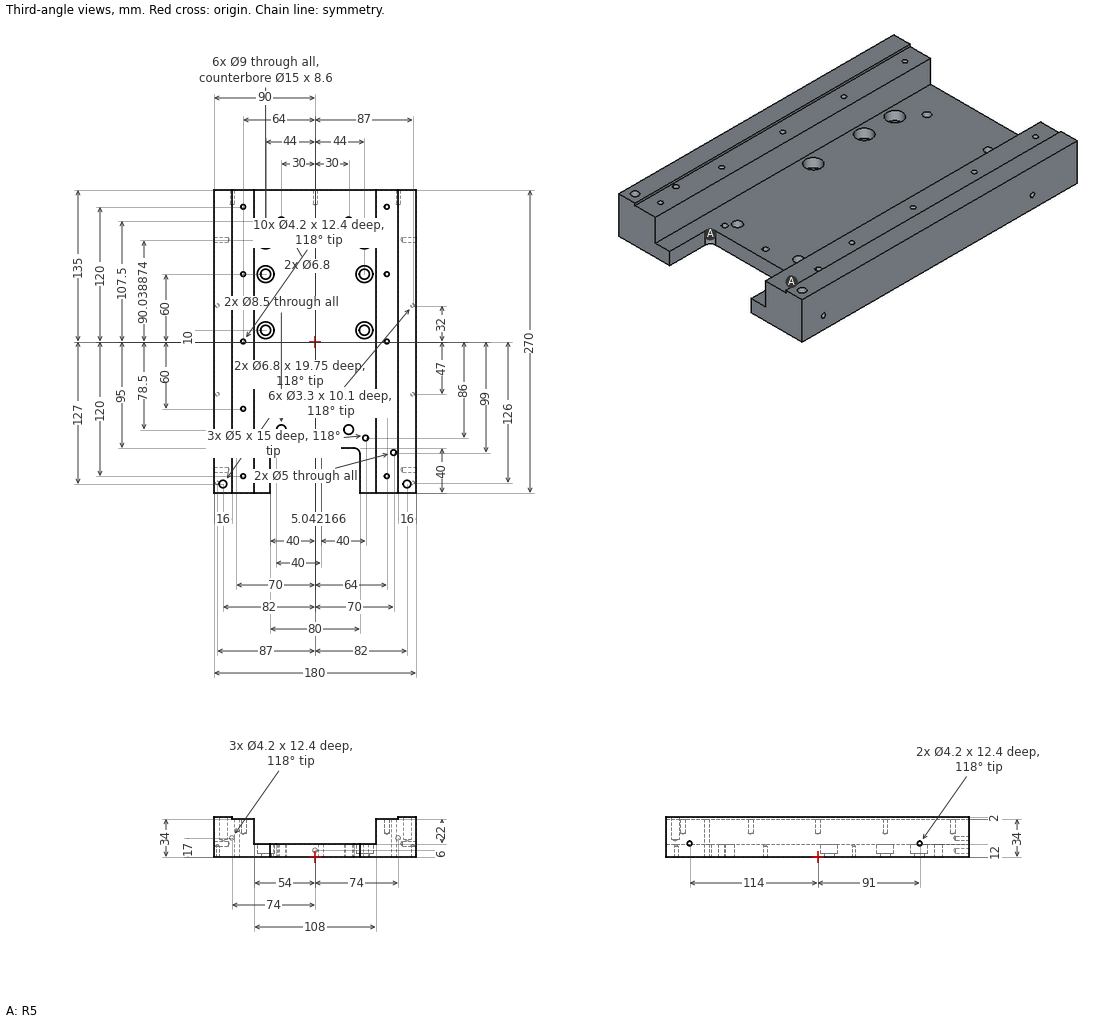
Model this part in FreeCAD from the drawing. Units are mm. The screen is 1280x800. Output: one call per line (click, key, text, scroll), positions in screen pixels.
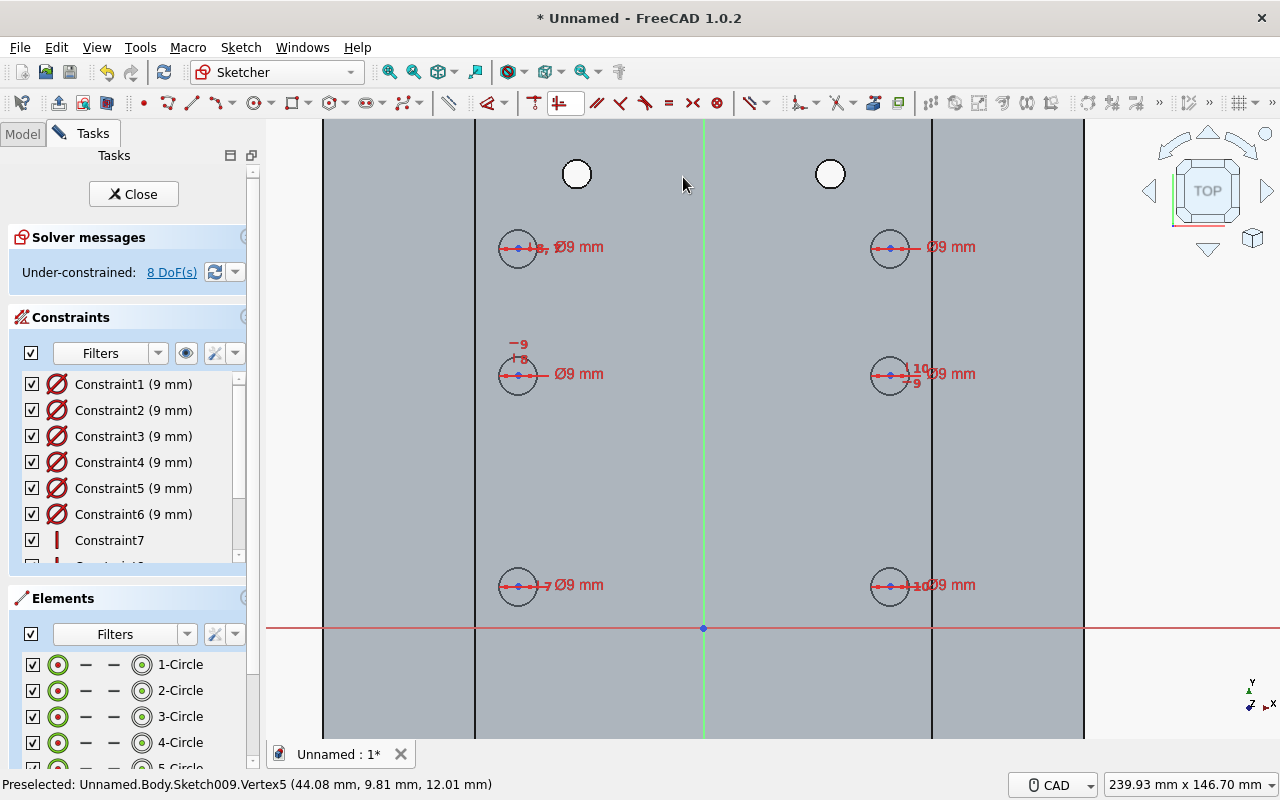
click(518, 587)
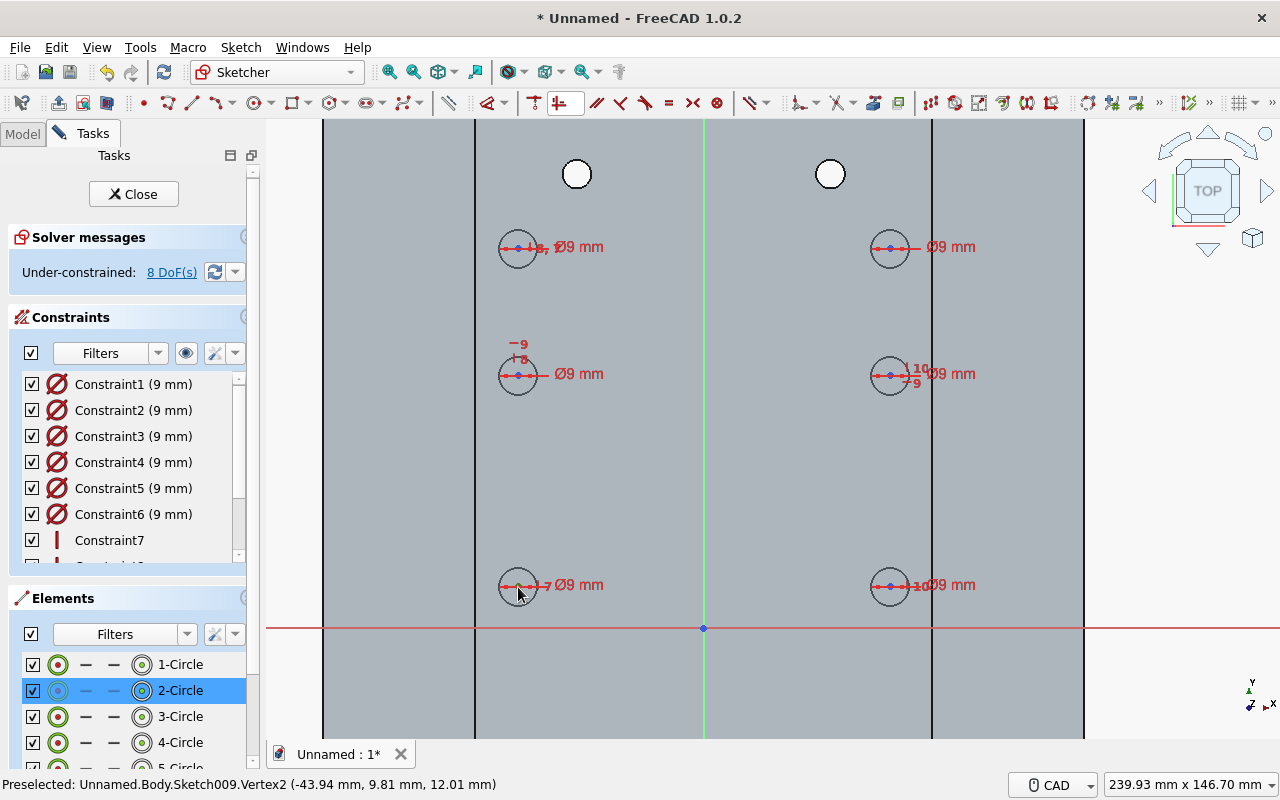
click(890, 587)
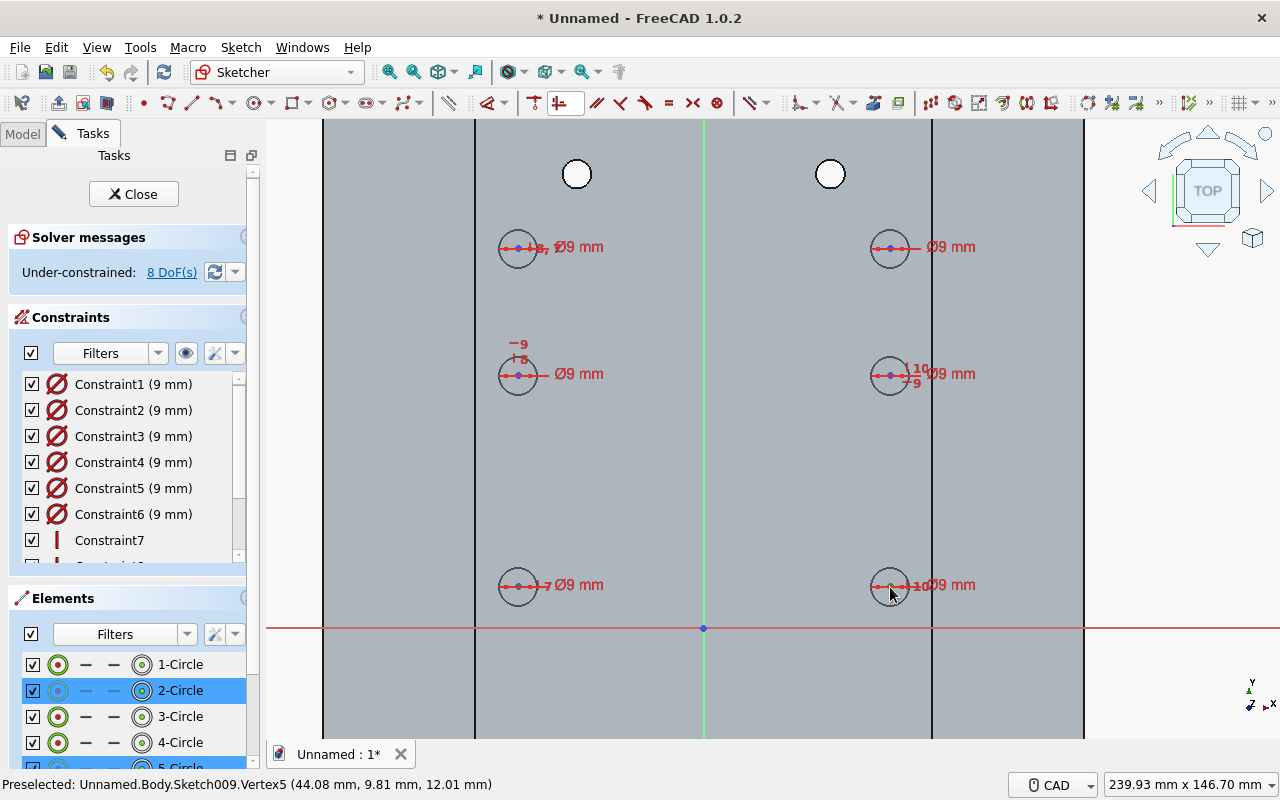
key(h)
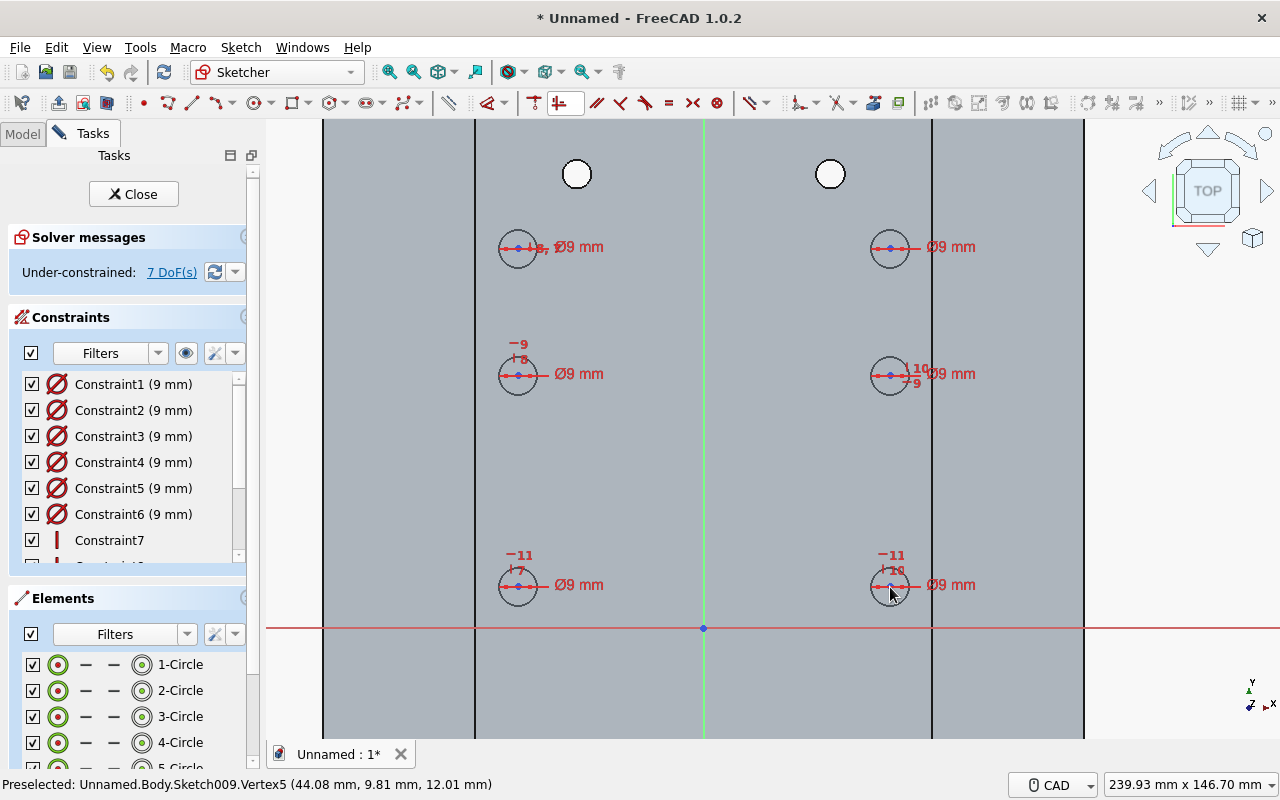
click(890, 376)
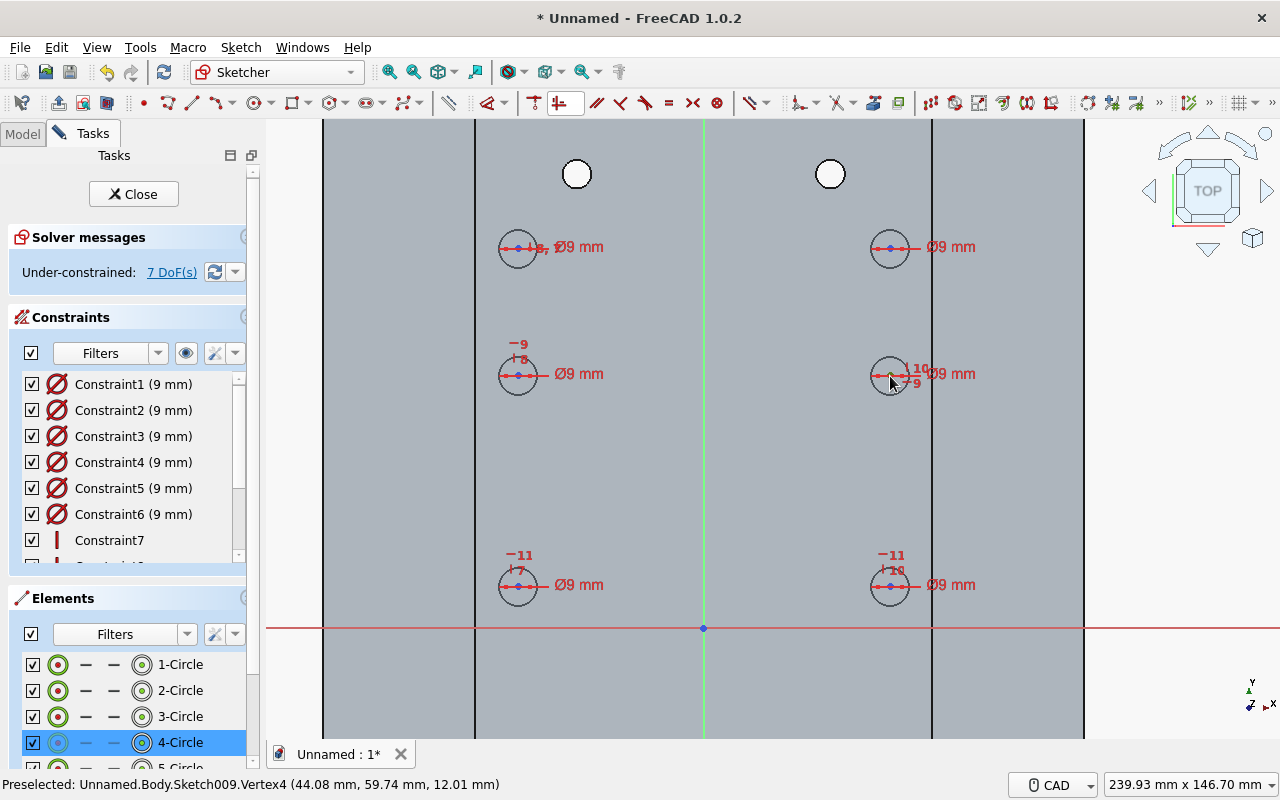
click(890, 249)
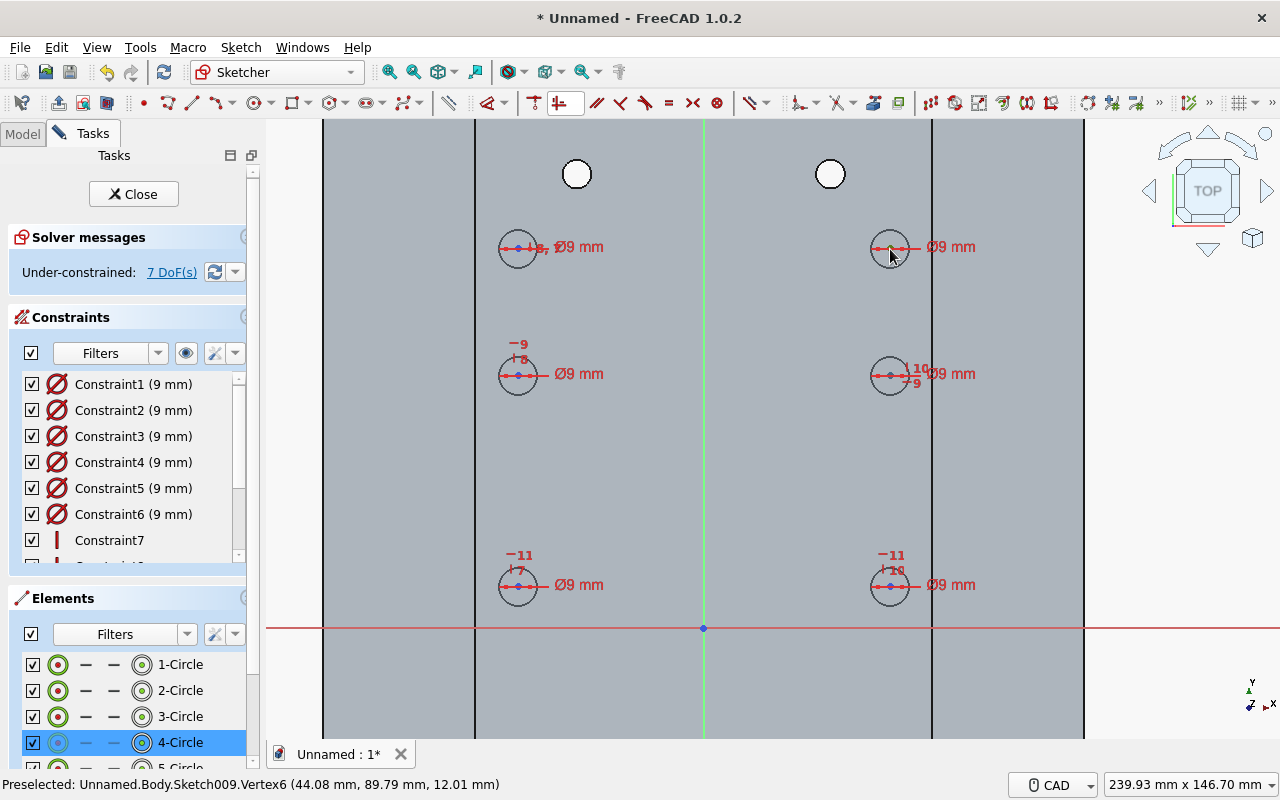
key(v)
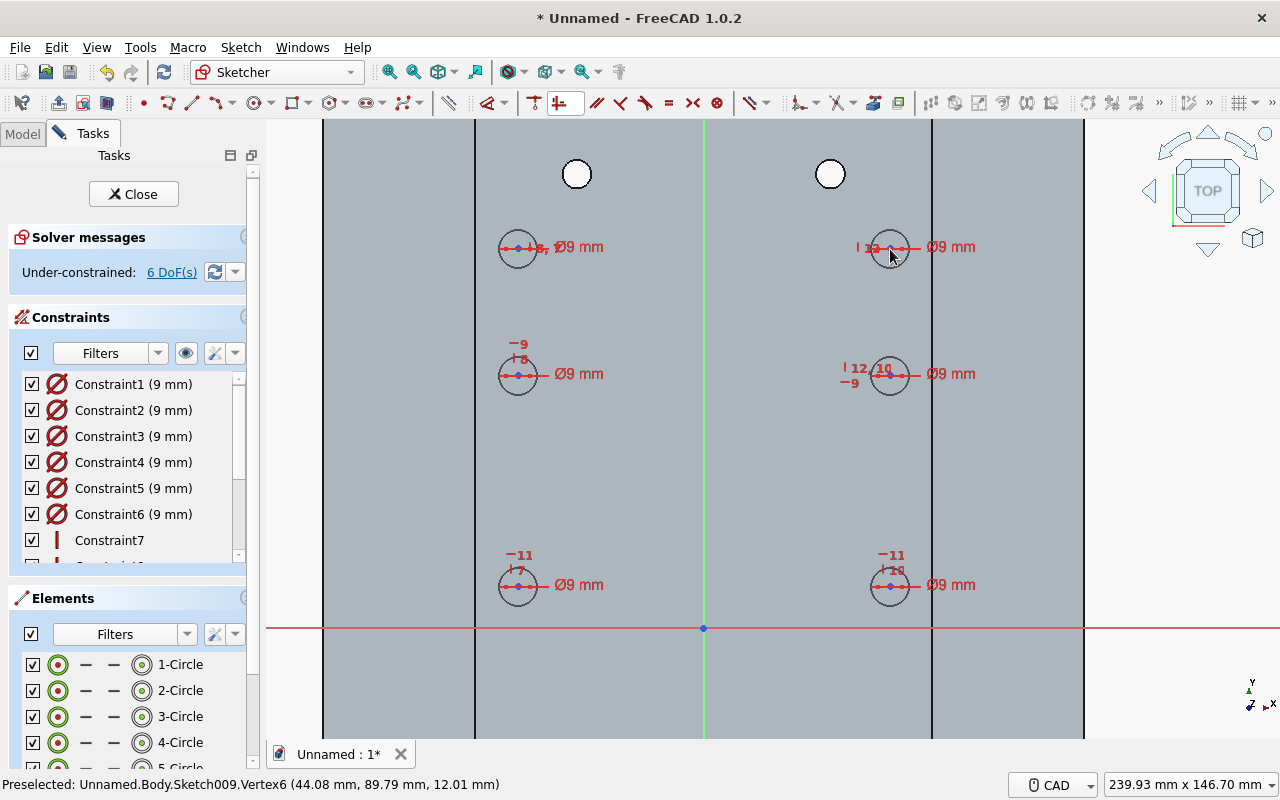
click(518, 249)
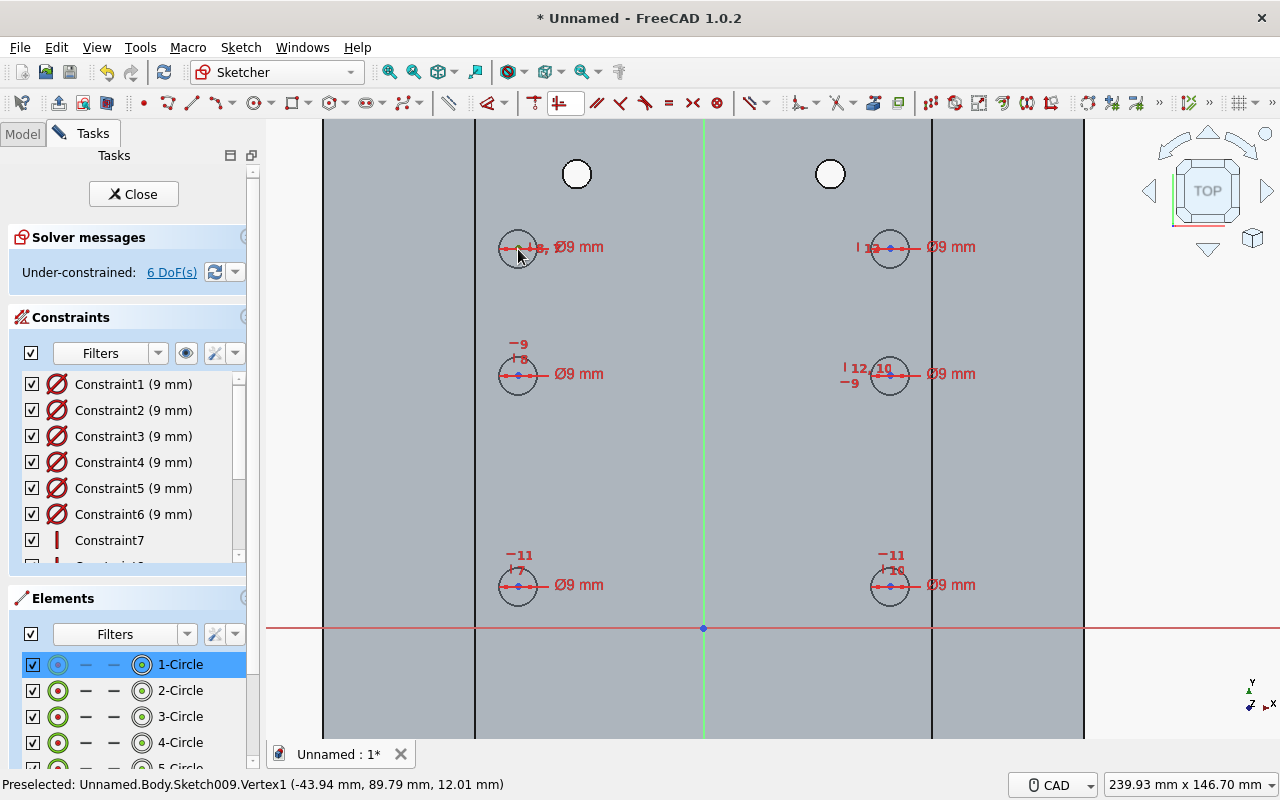
click(890, 249)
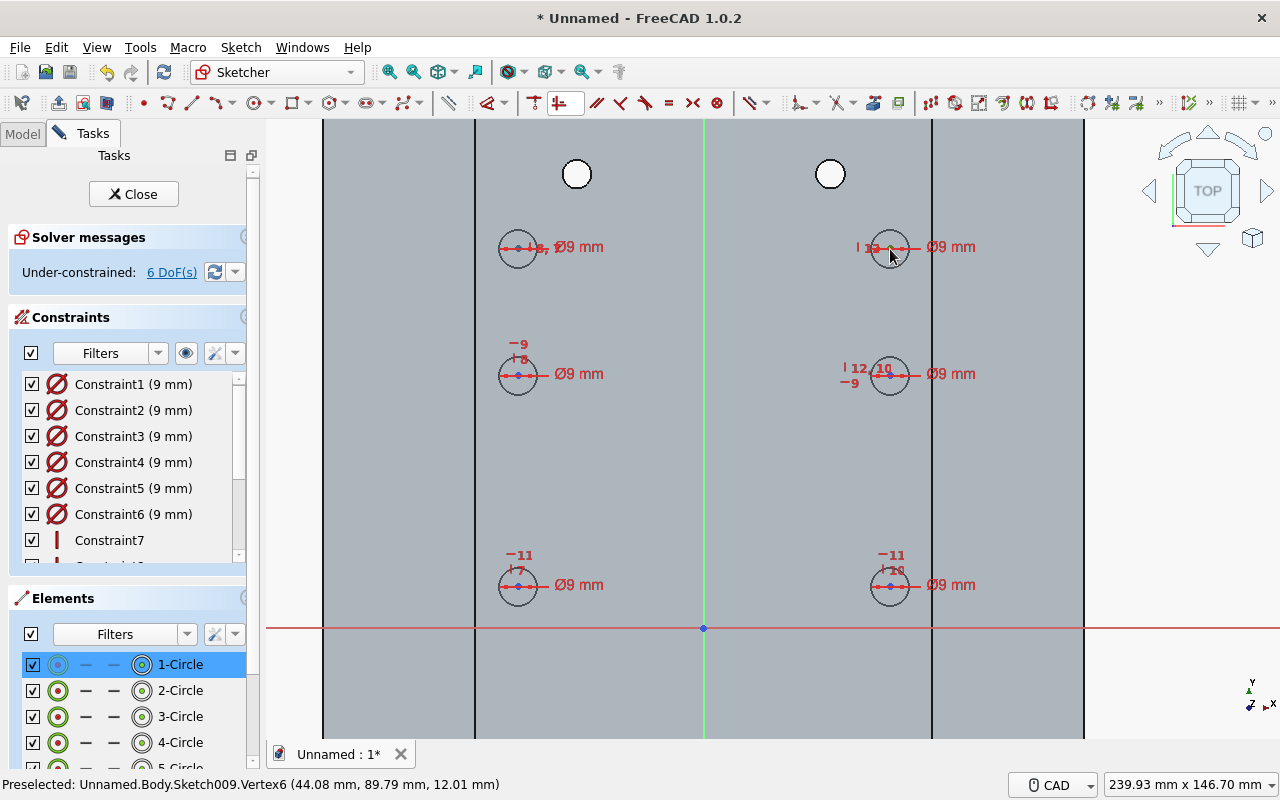
click(578, 104)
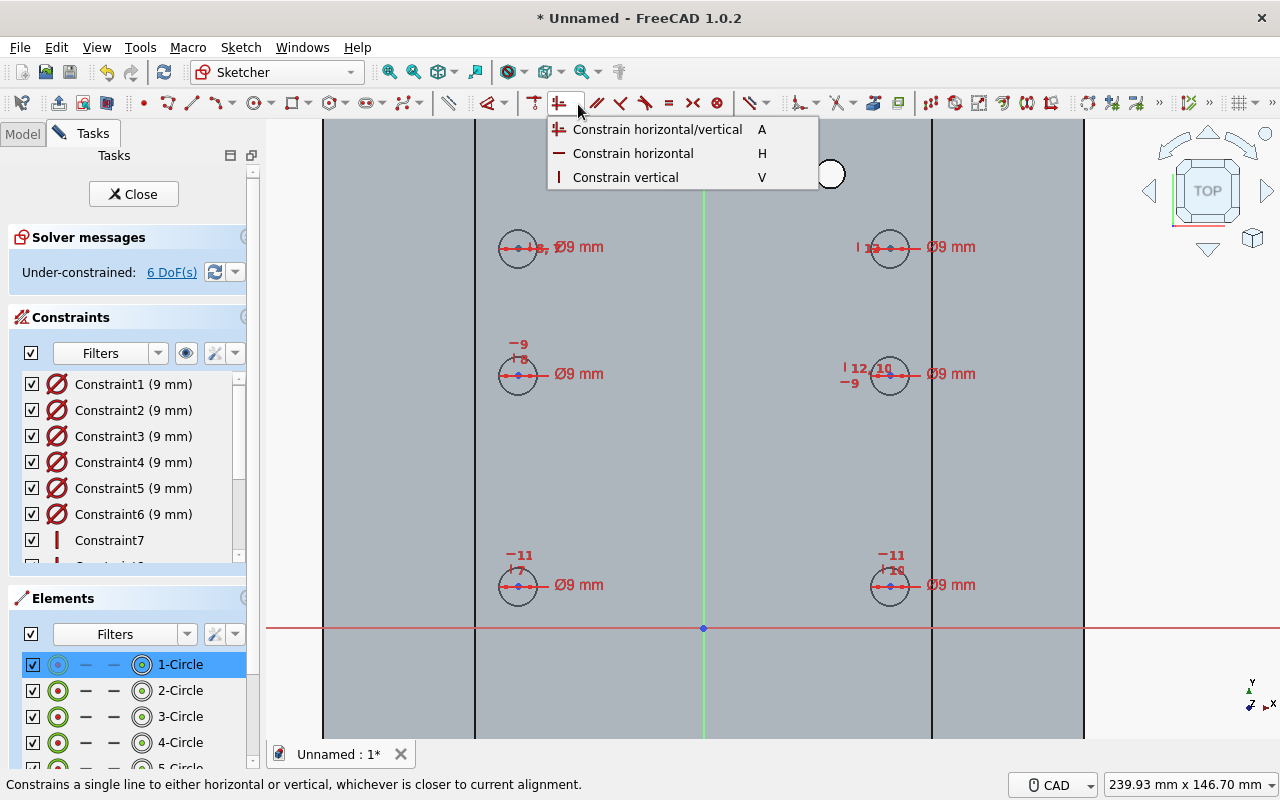
click(683, 153)